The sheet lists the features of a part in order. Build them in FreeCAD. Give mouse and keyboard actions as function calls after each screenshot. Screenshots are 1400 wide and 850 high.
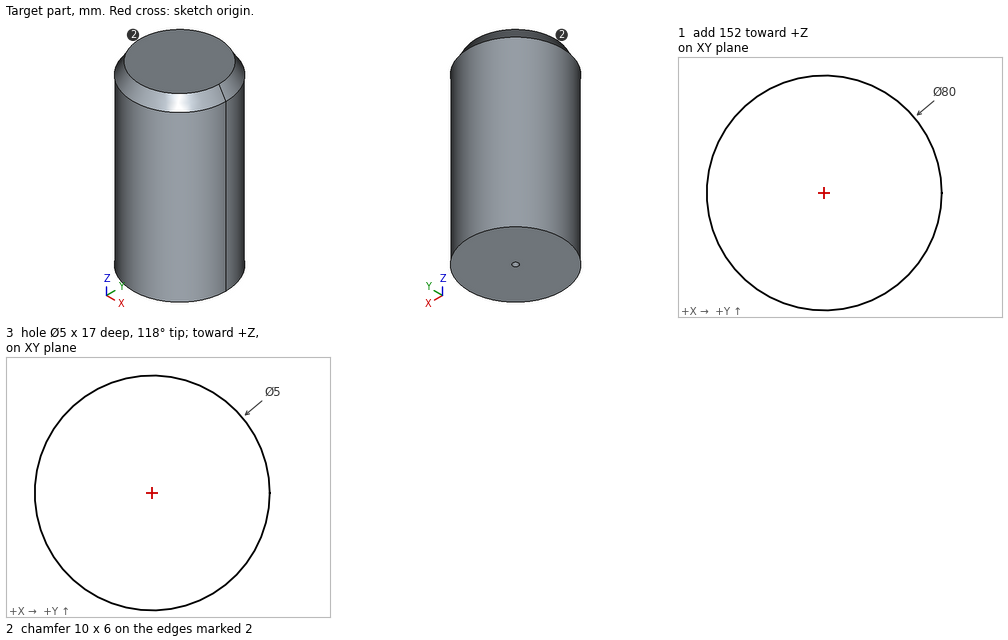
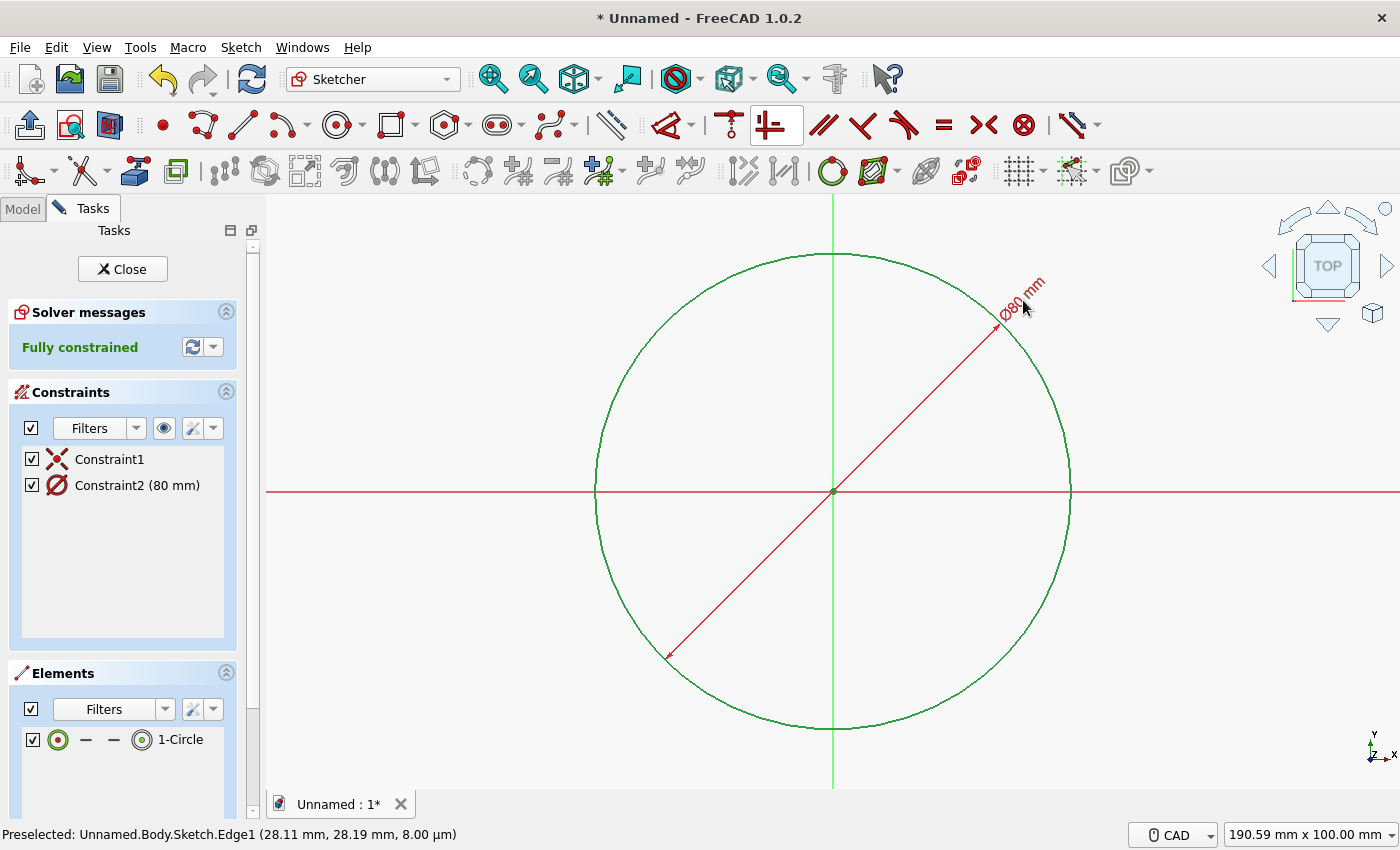
click(123, 269)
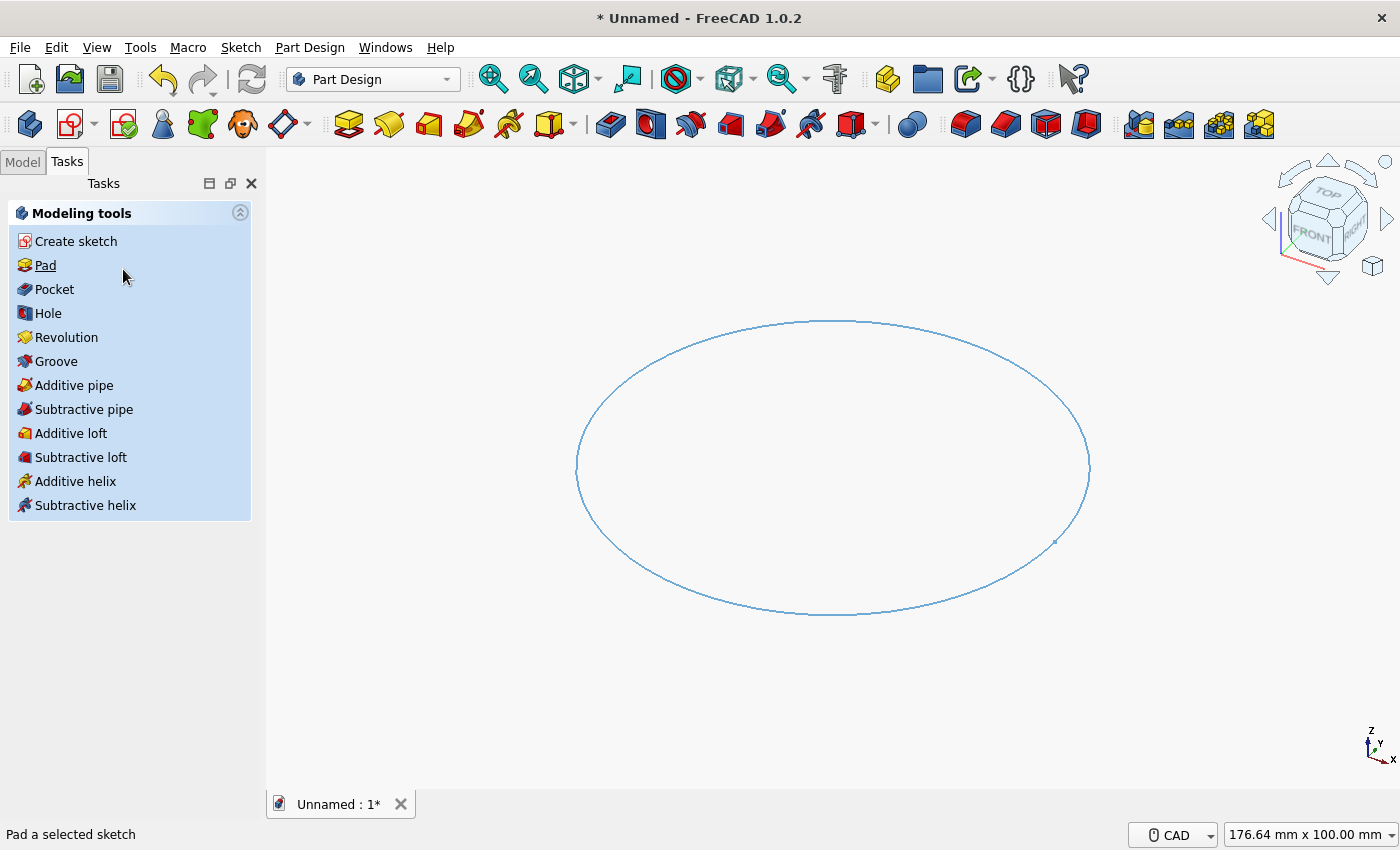
click(350, 124)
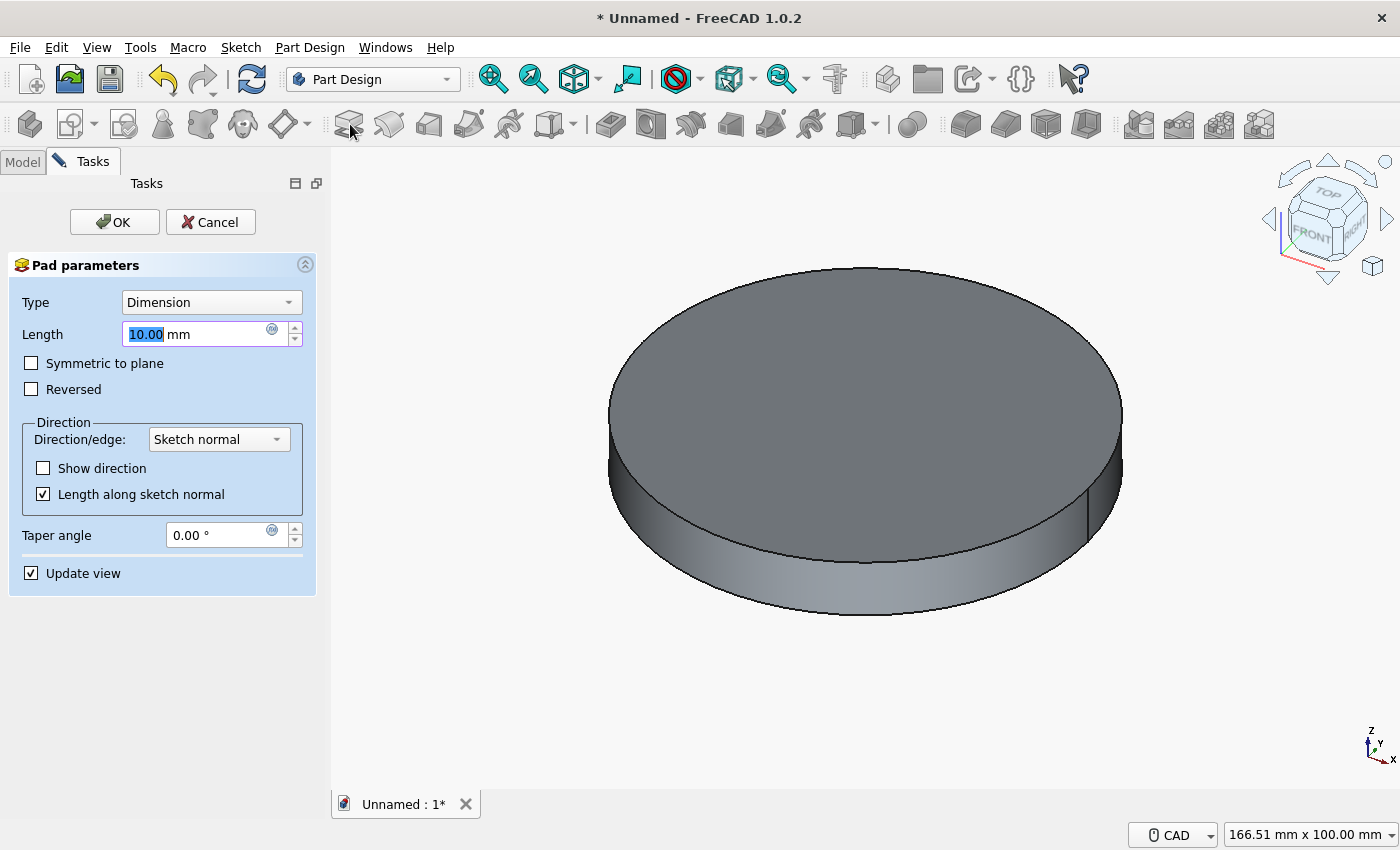
text(152)
key(Tab)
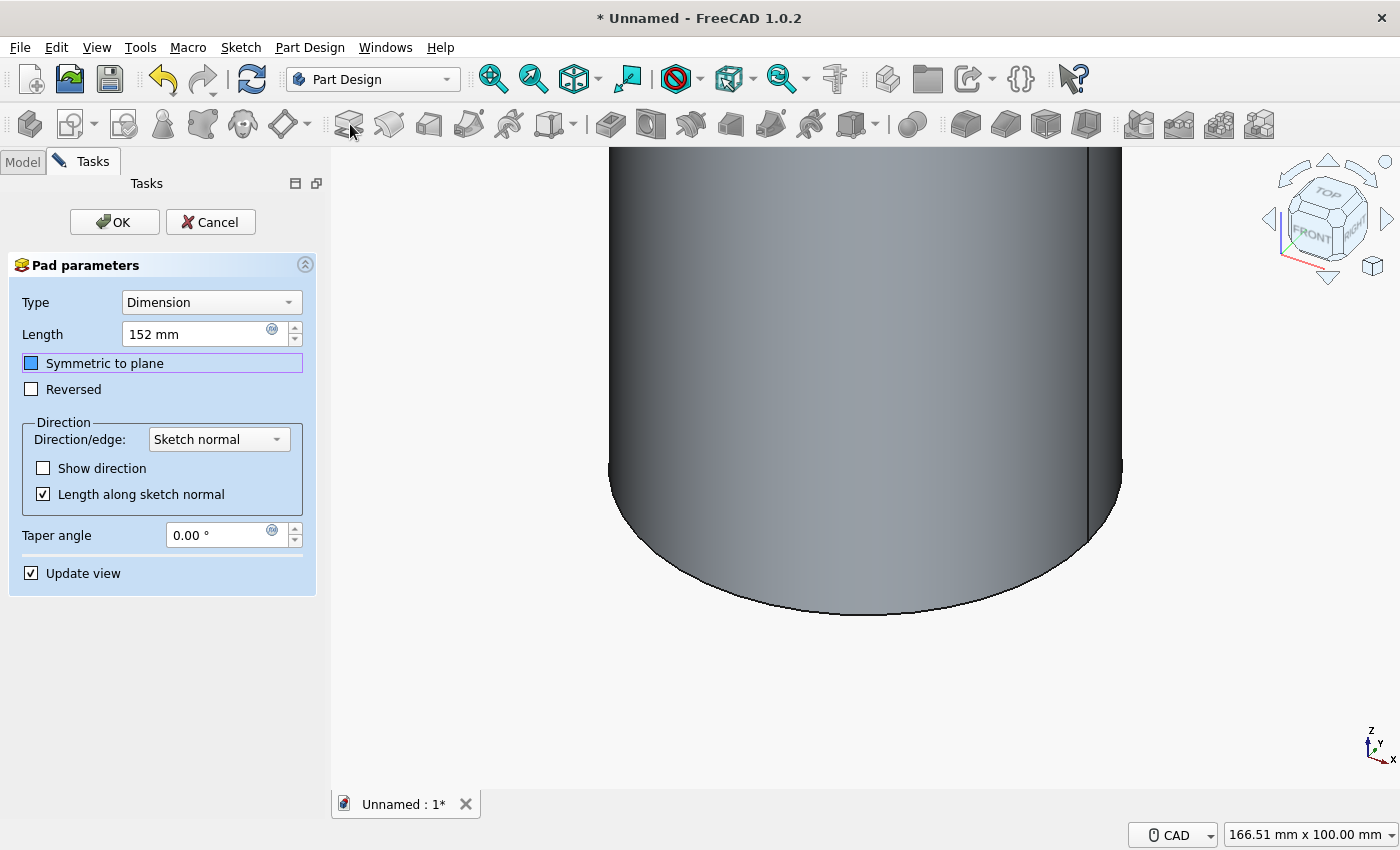
click(115, 222)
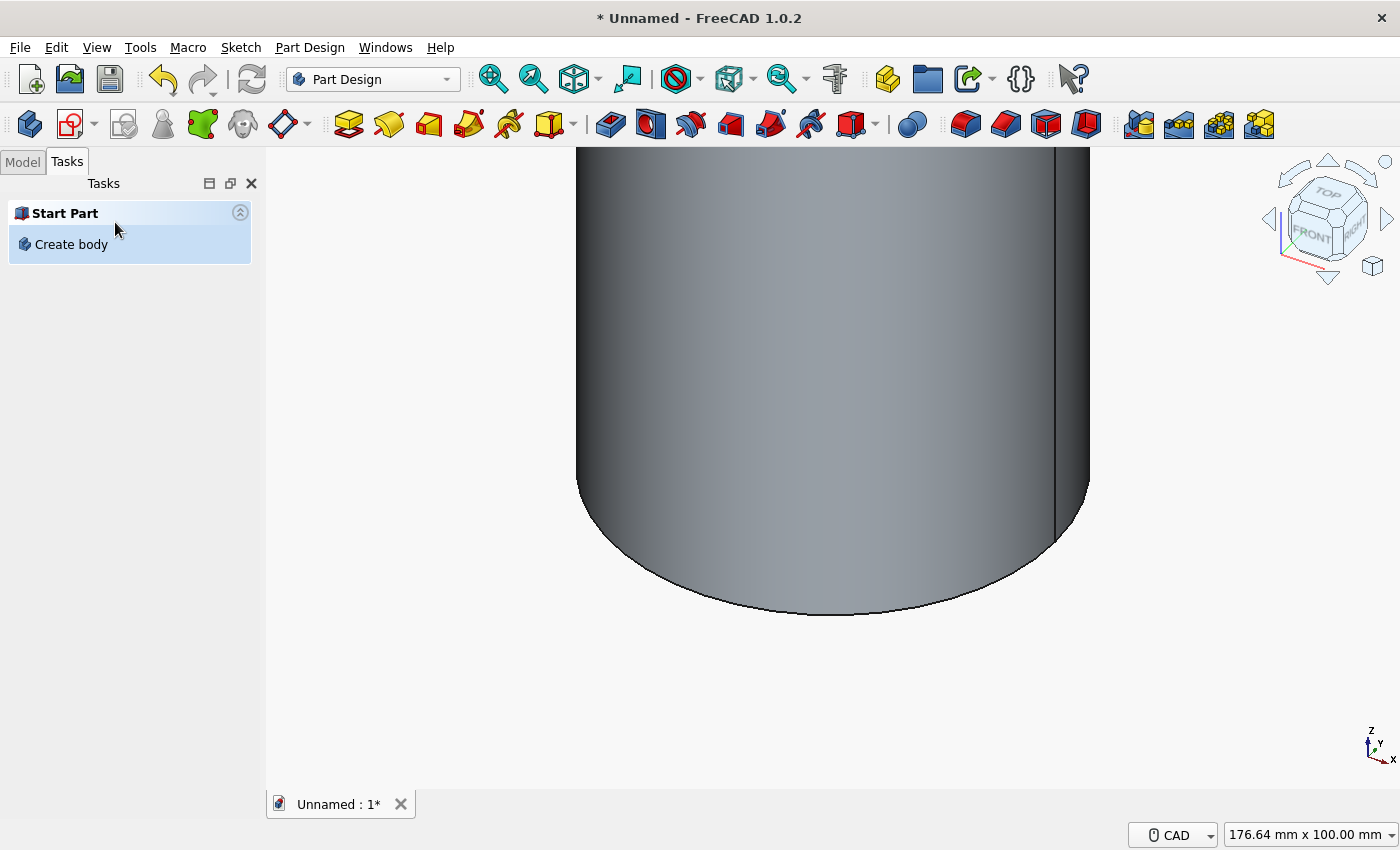
click(494, 80)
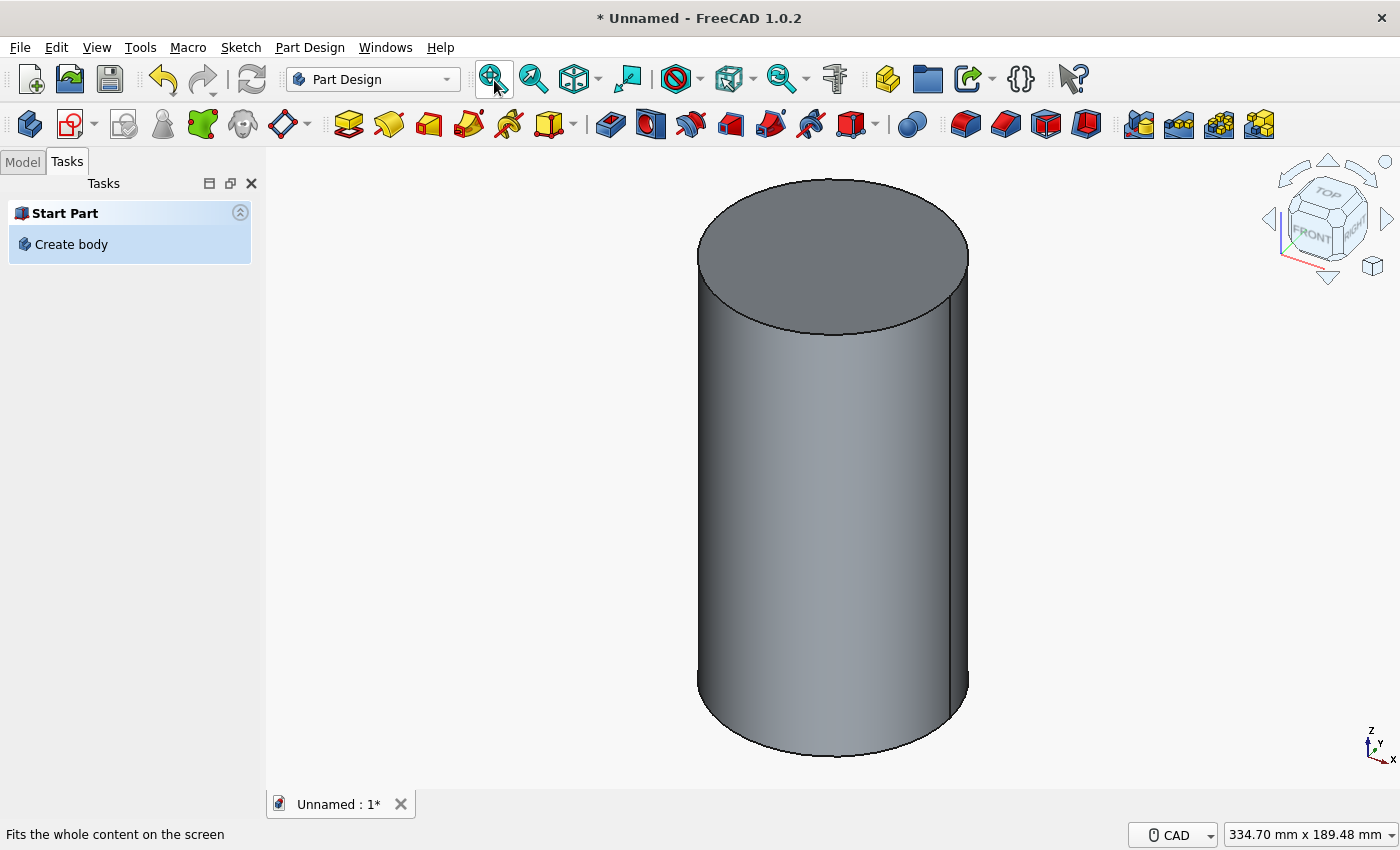
click(698, 264)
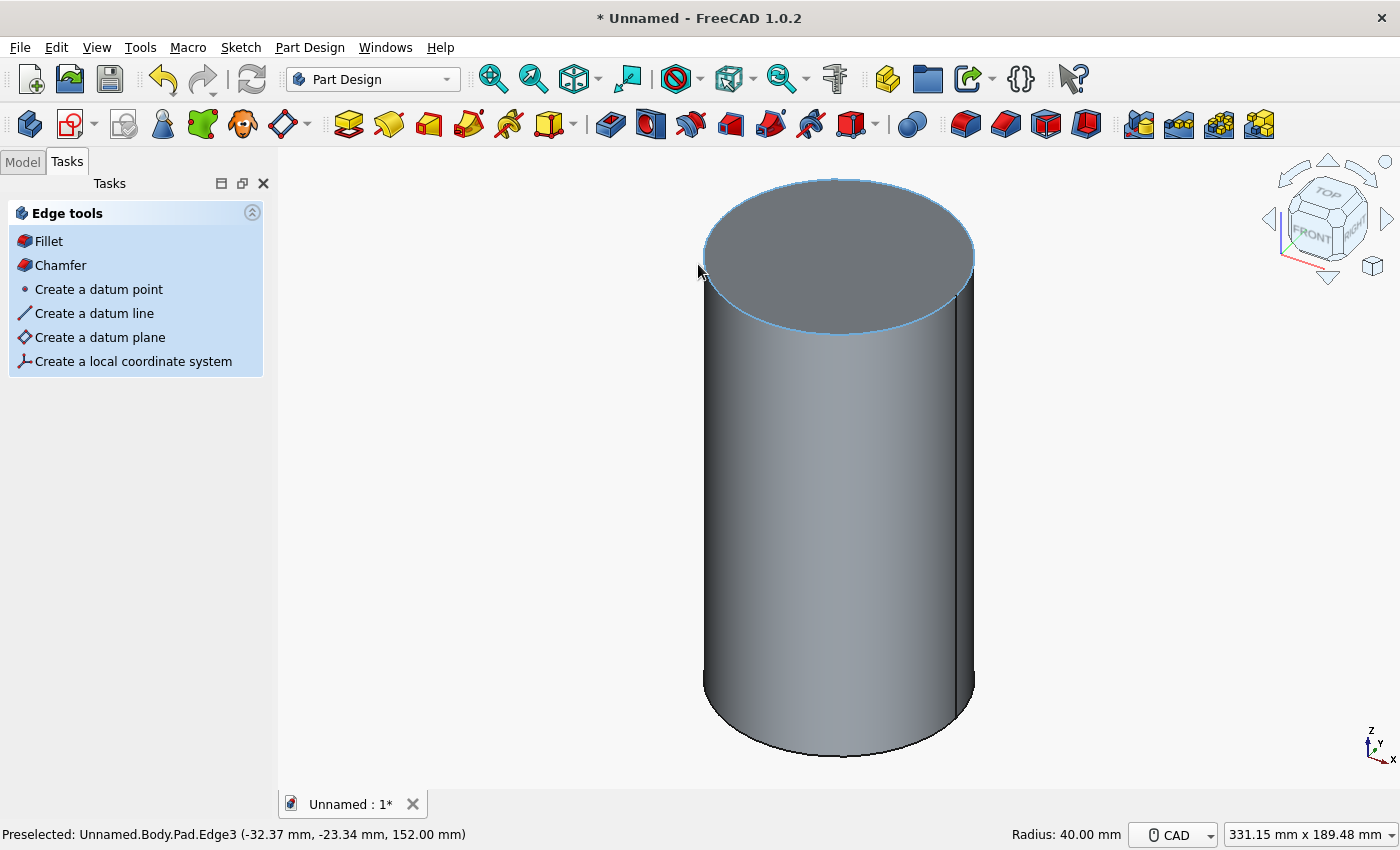
click(1006, 124)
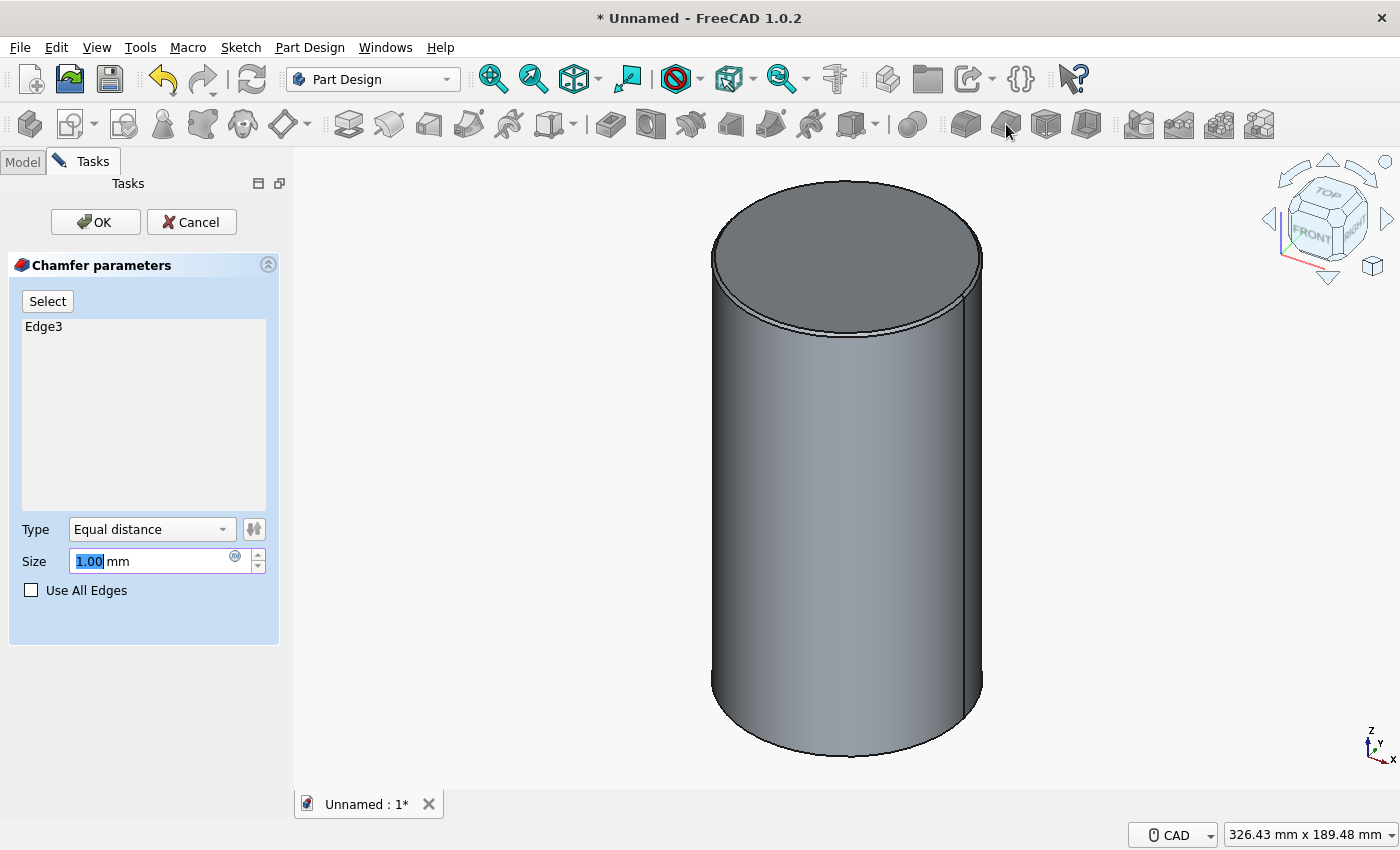
text(10)
key(Tab)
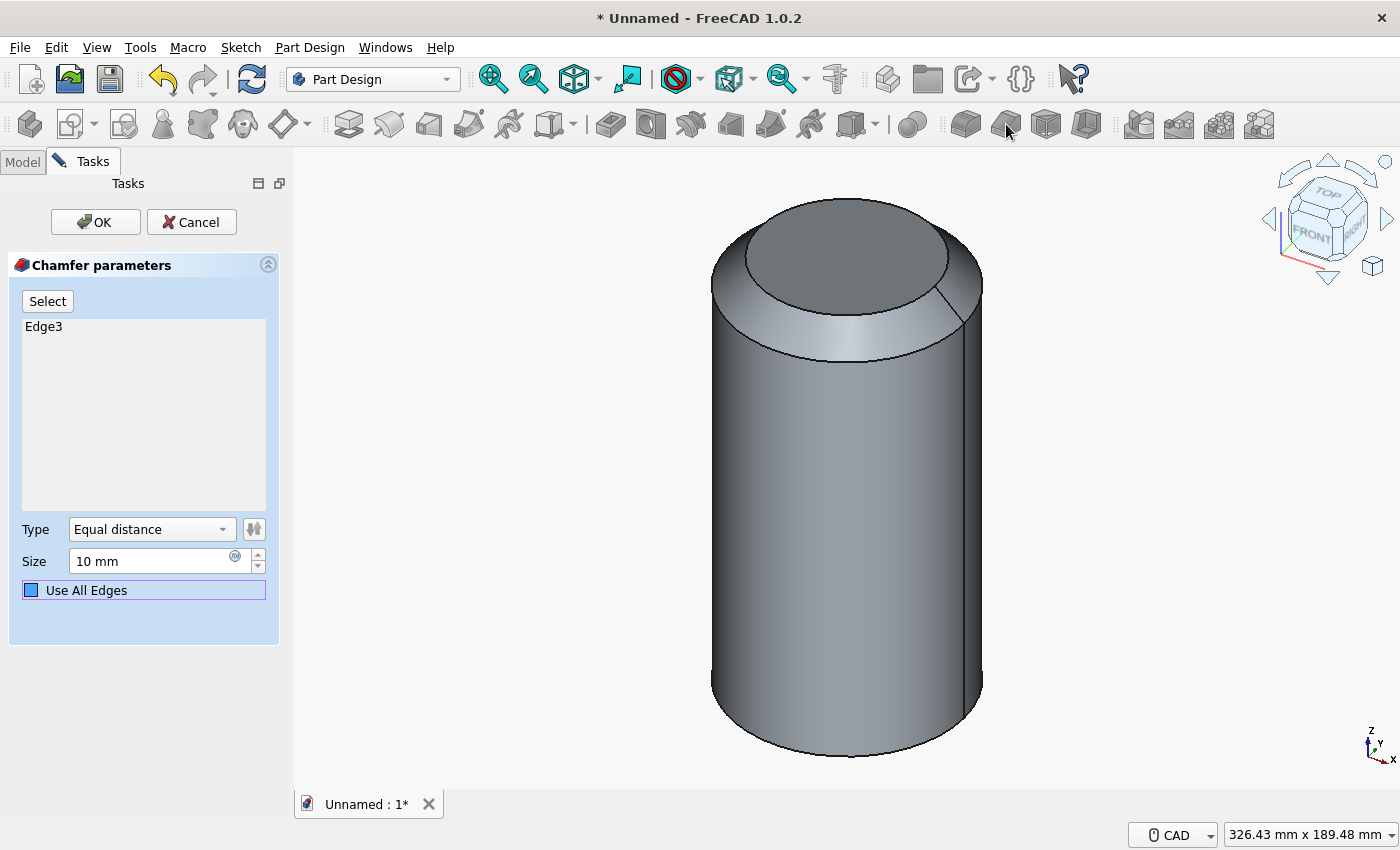
click(153, 530)